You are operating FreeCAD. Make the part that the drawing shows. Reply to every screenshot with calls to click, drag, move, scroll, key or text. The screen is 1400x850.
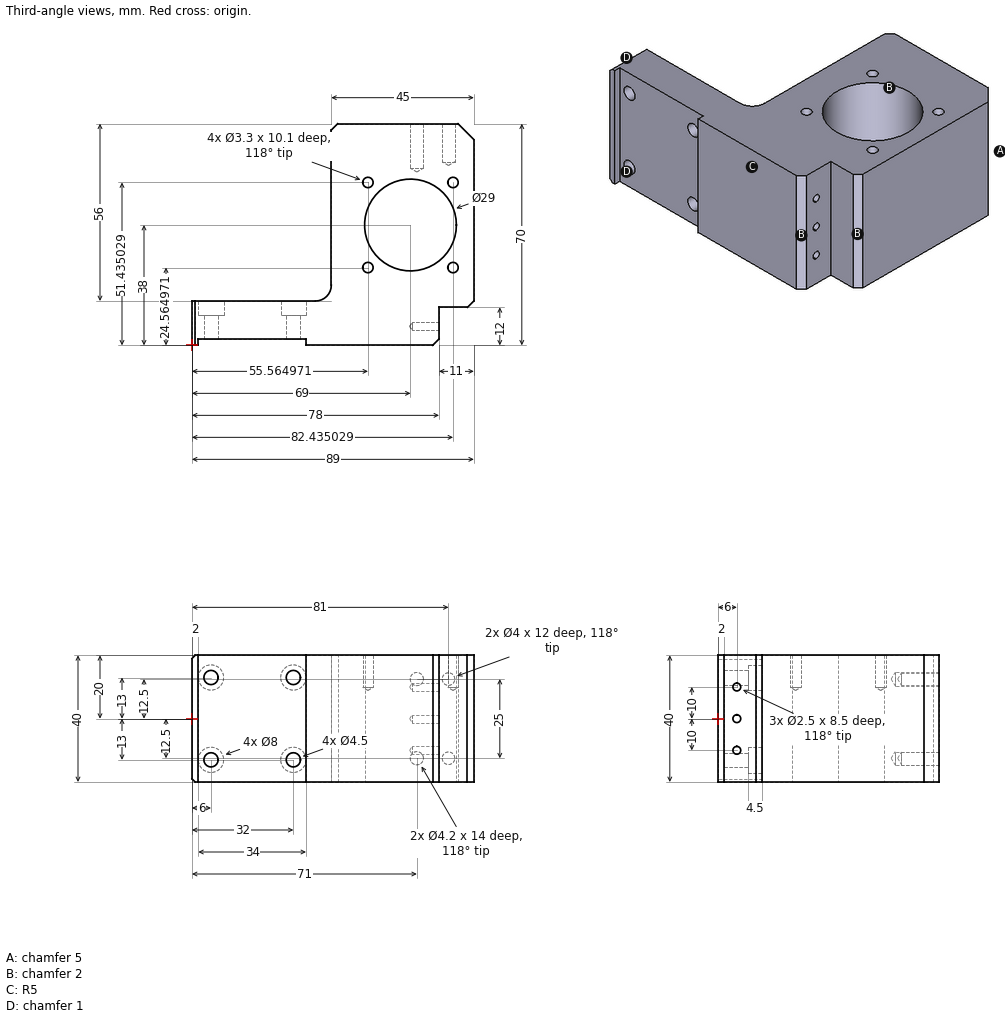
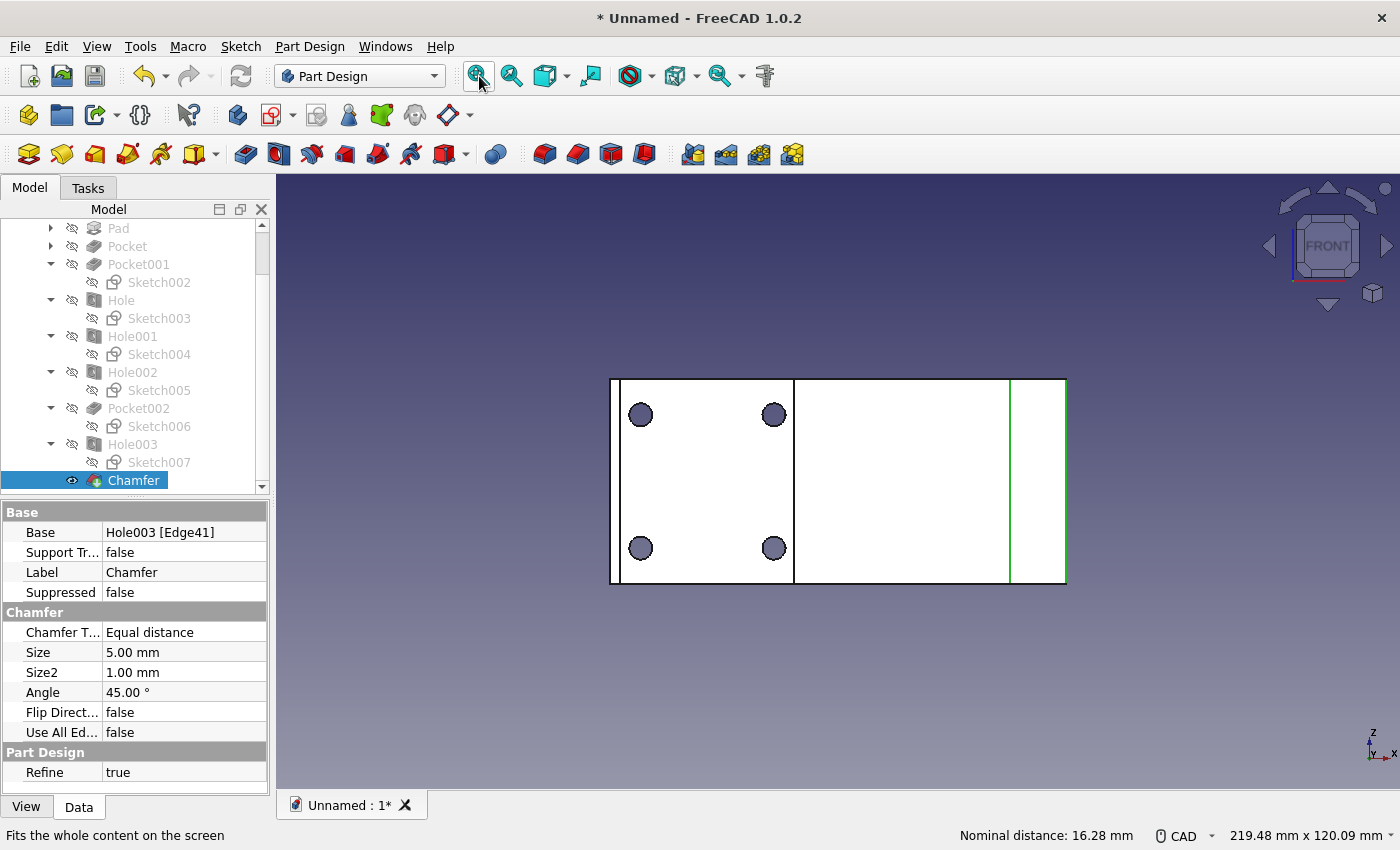
key(3)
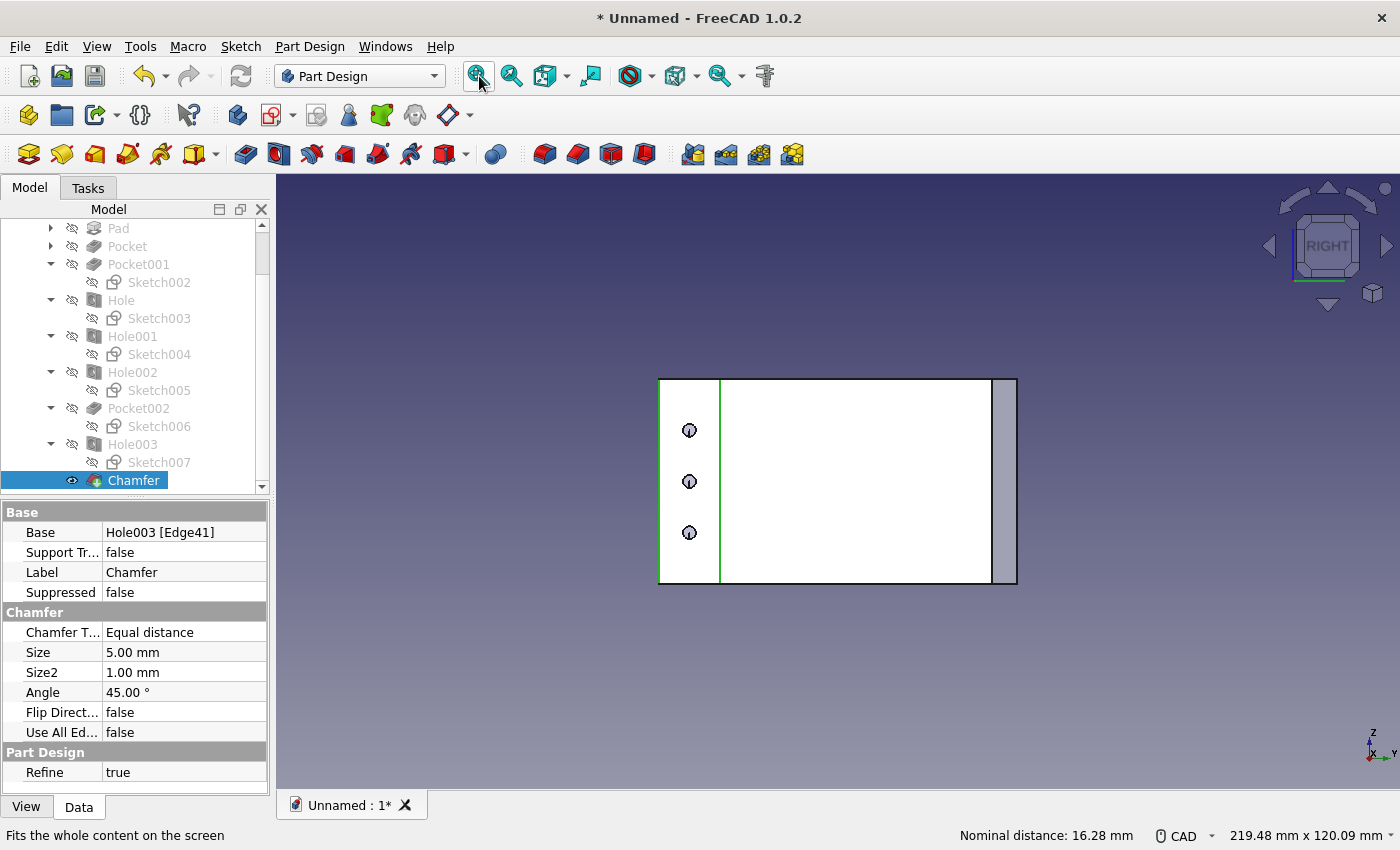
key(v)
key(f)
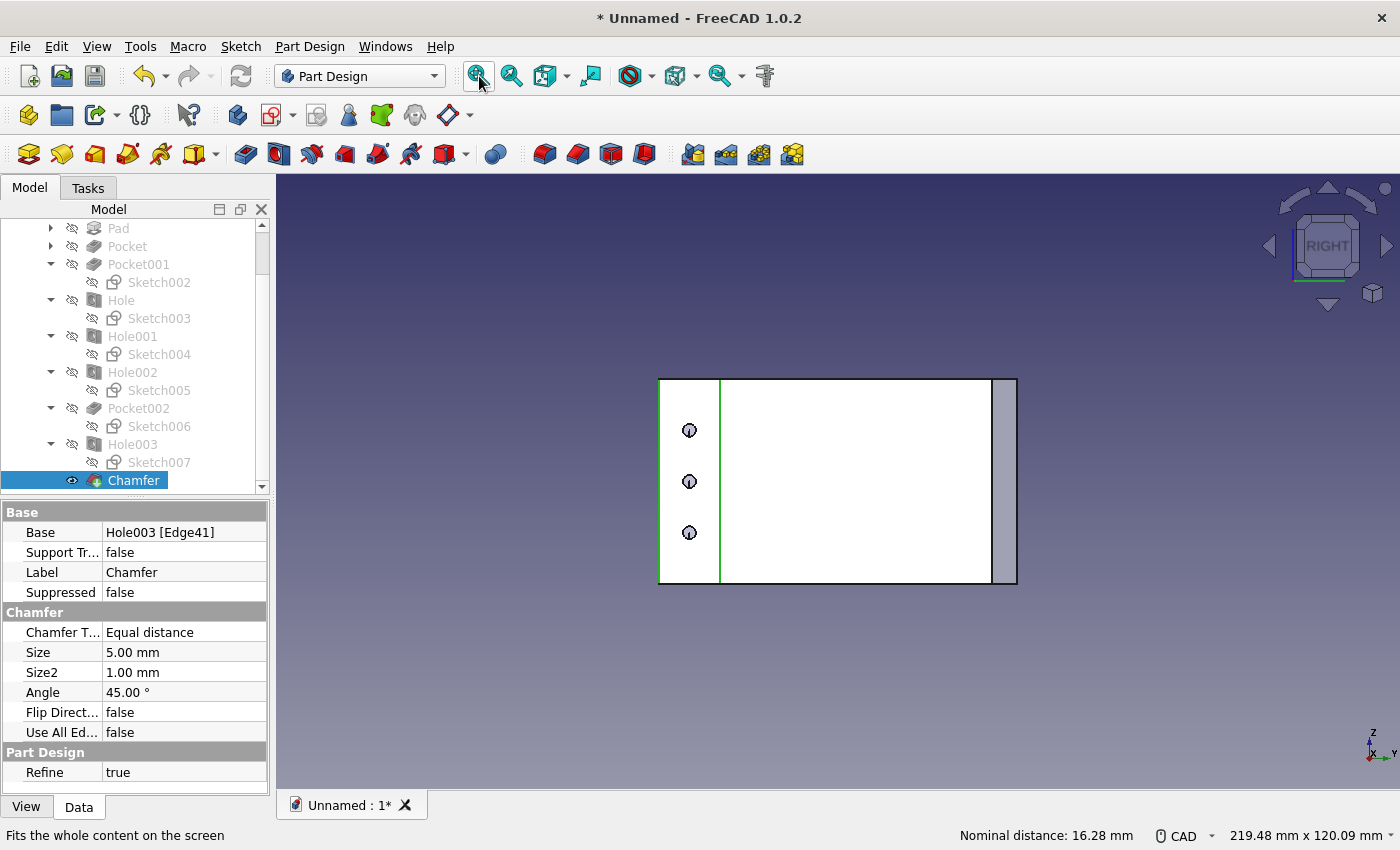
key(5)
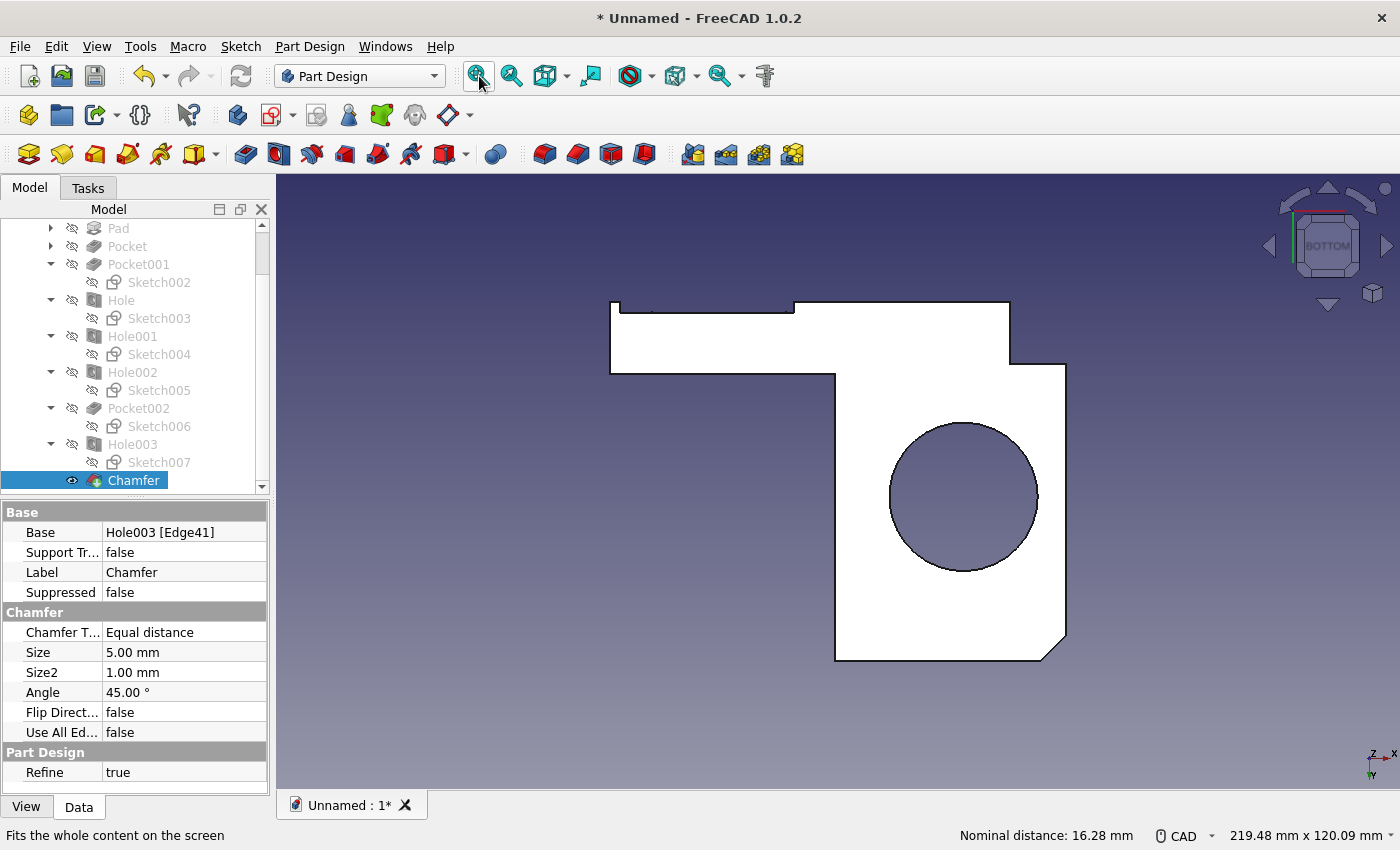
key(4)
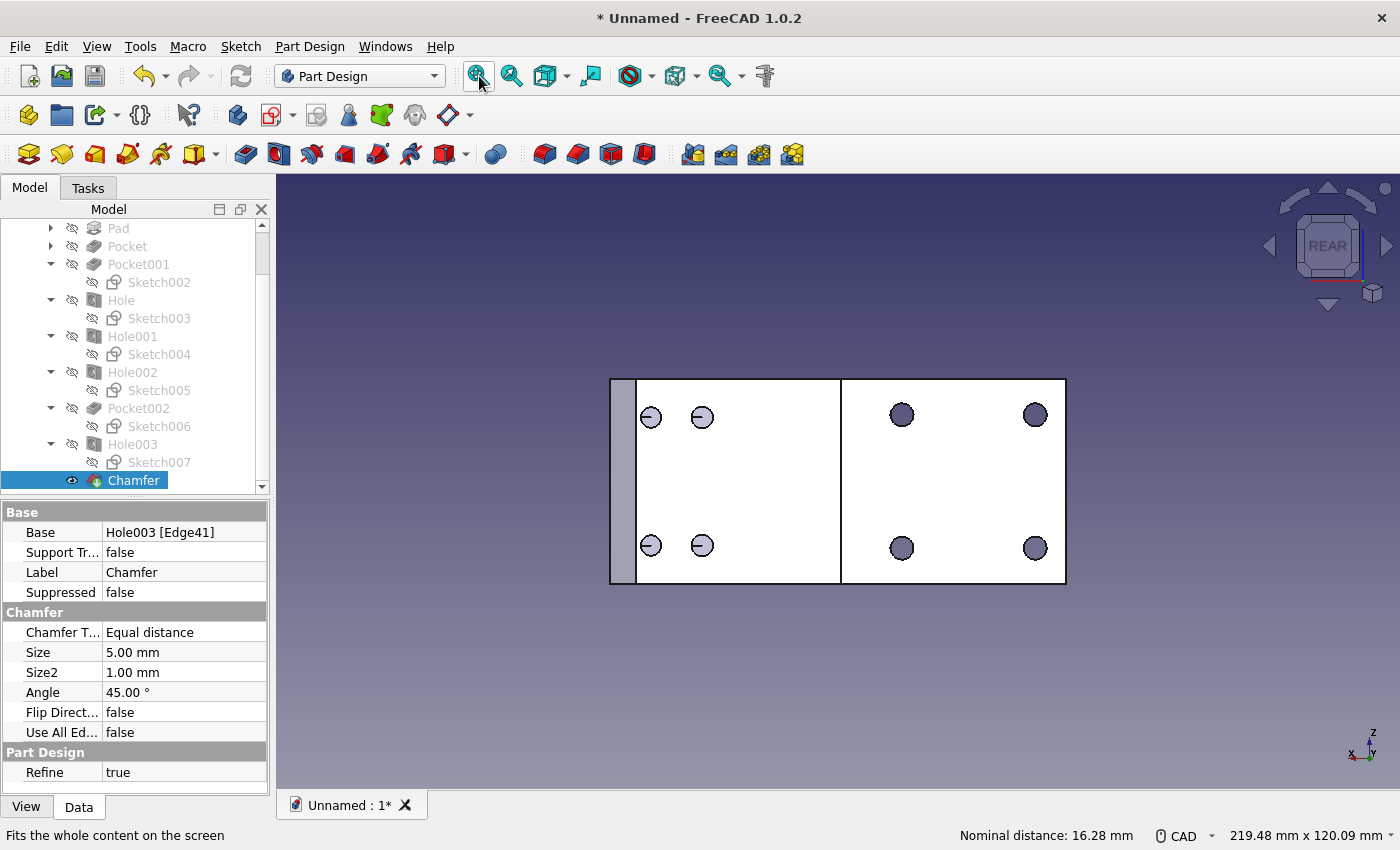
click(479, 76)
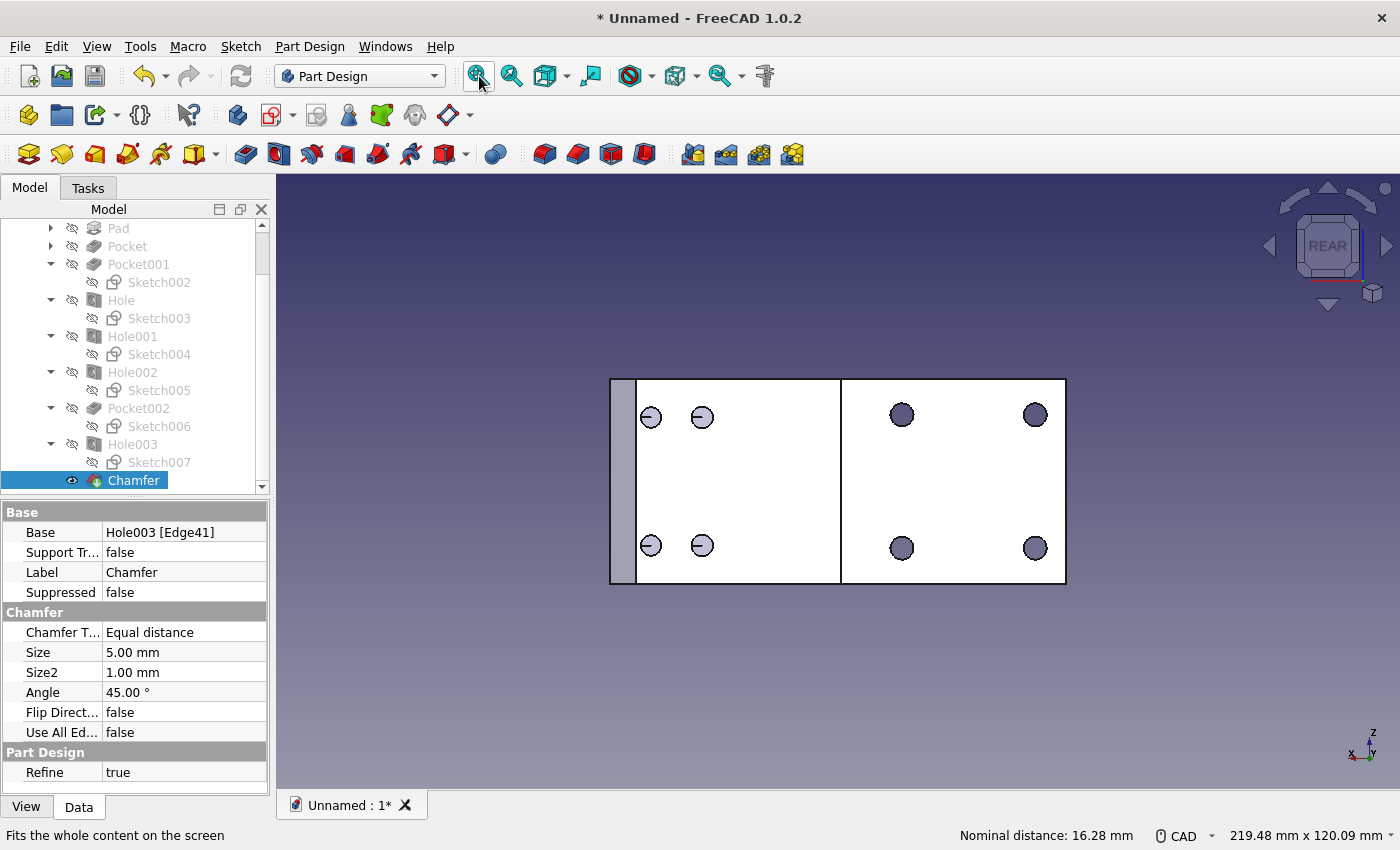
click(841, 481, ctrl)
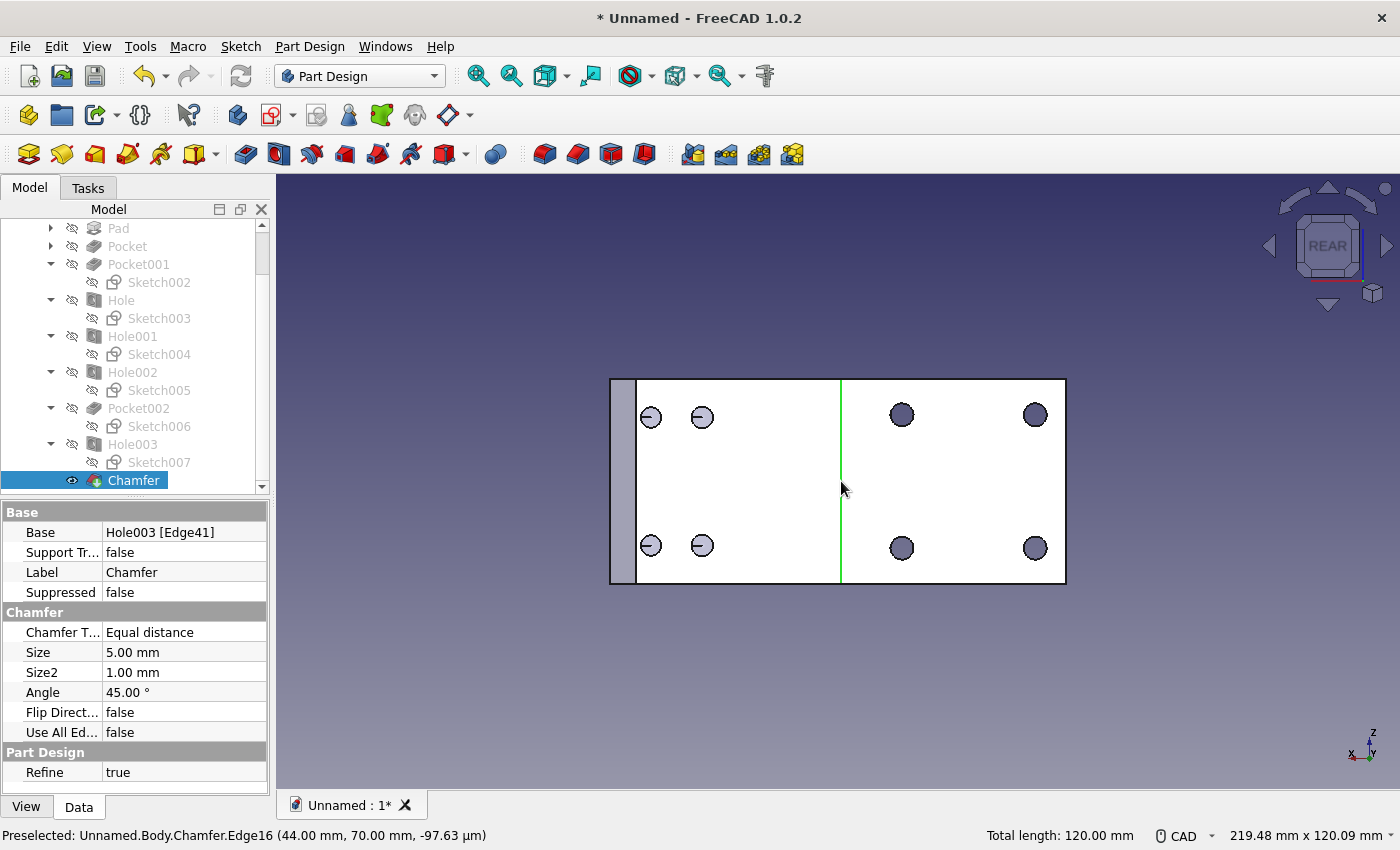
click(578, 154)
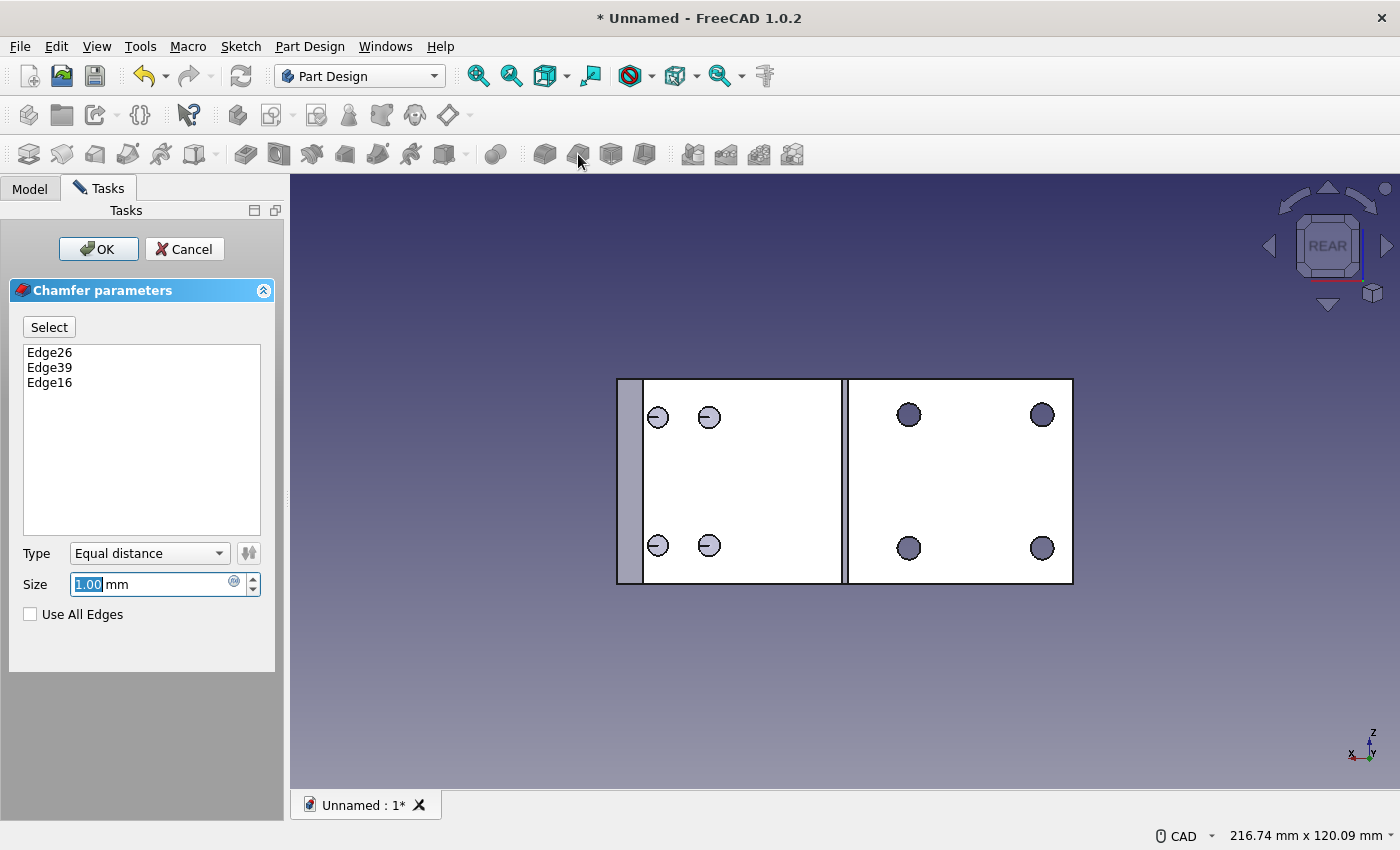
text(2)
key(Tab)